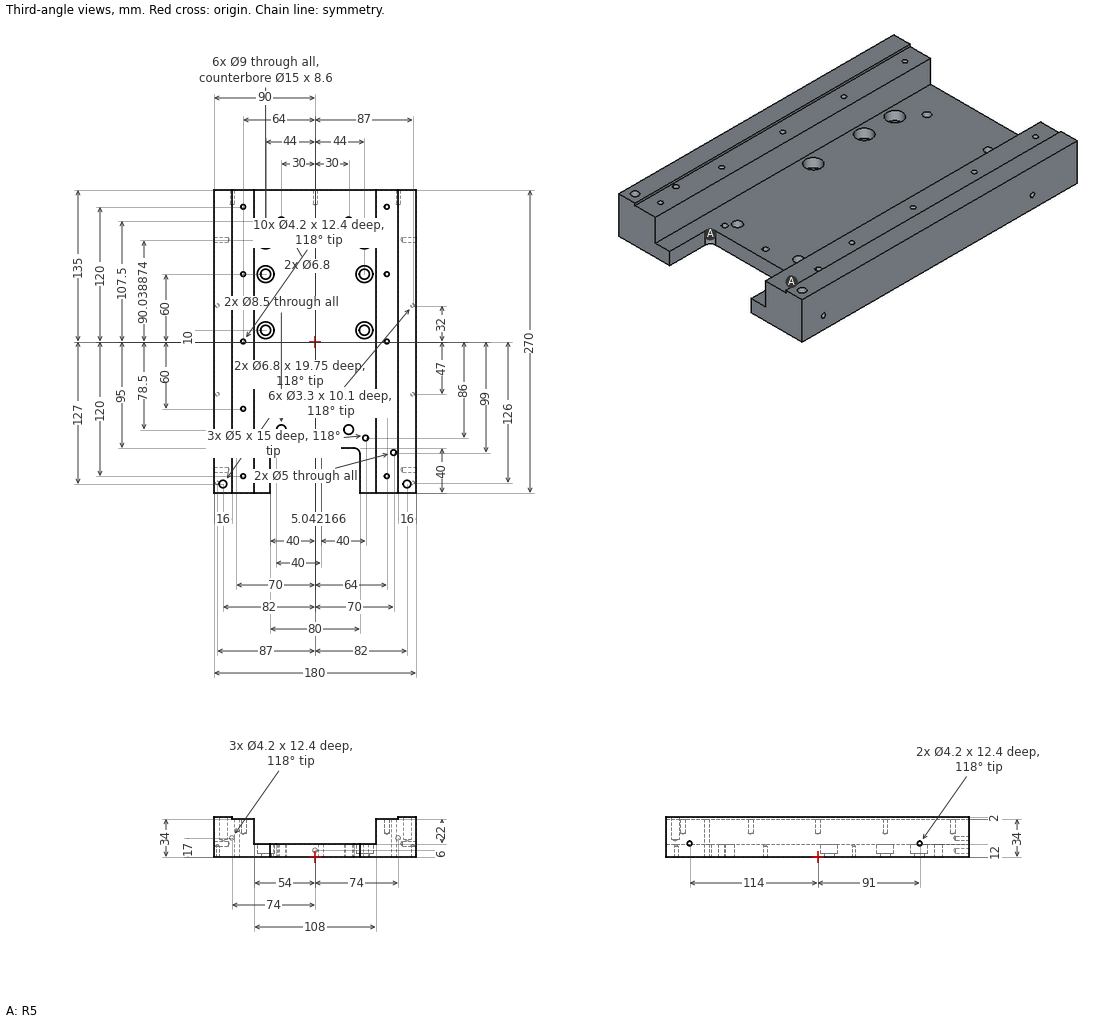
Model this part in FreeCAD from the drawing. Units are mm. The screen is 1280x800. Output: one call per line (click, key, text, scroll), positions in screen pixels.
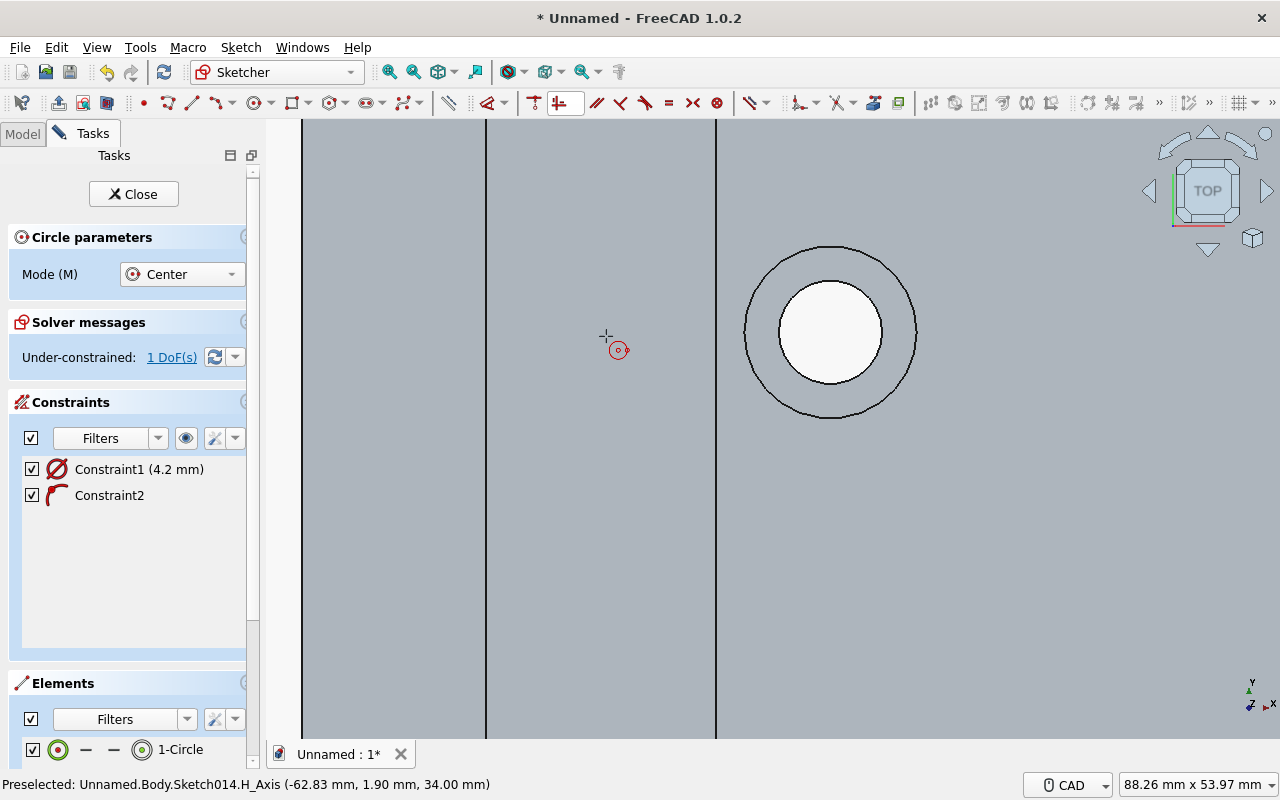
scroll(606, 336, down, 10)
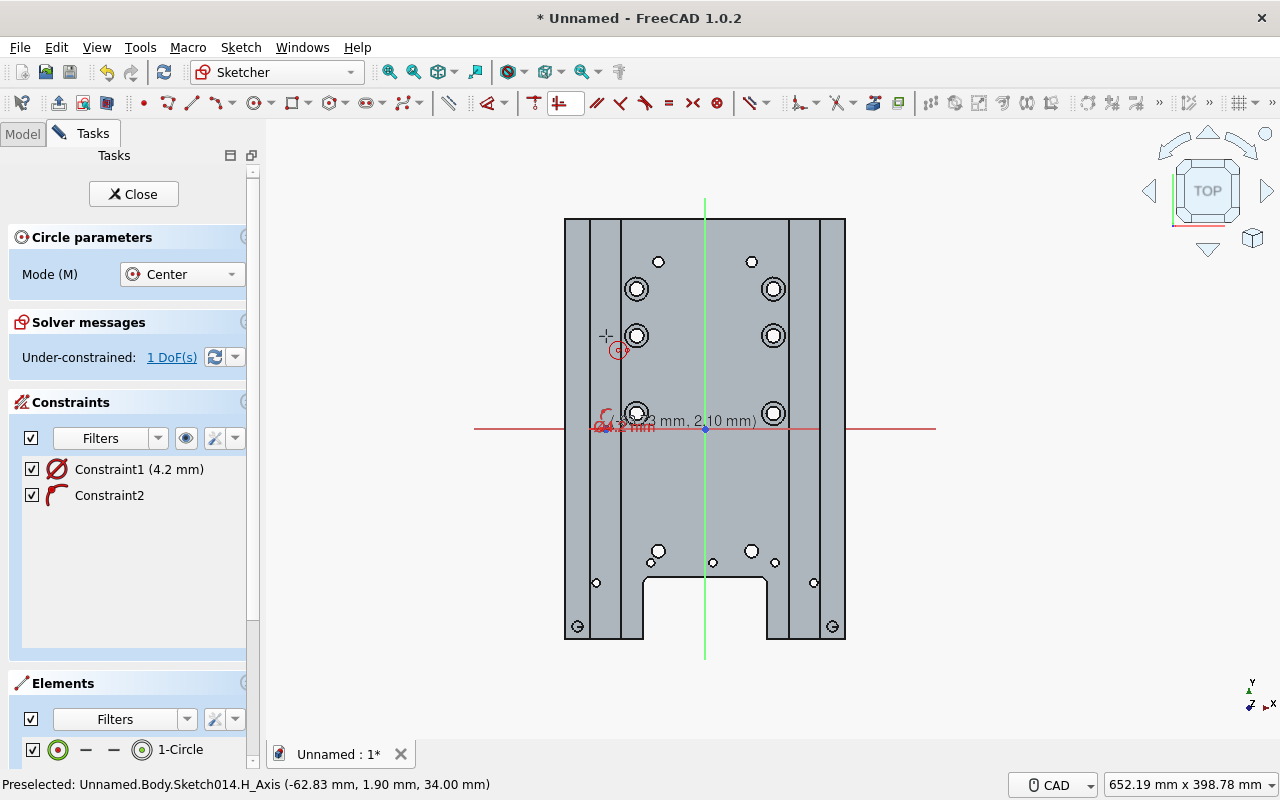
click(606, 336)
move(608, 333)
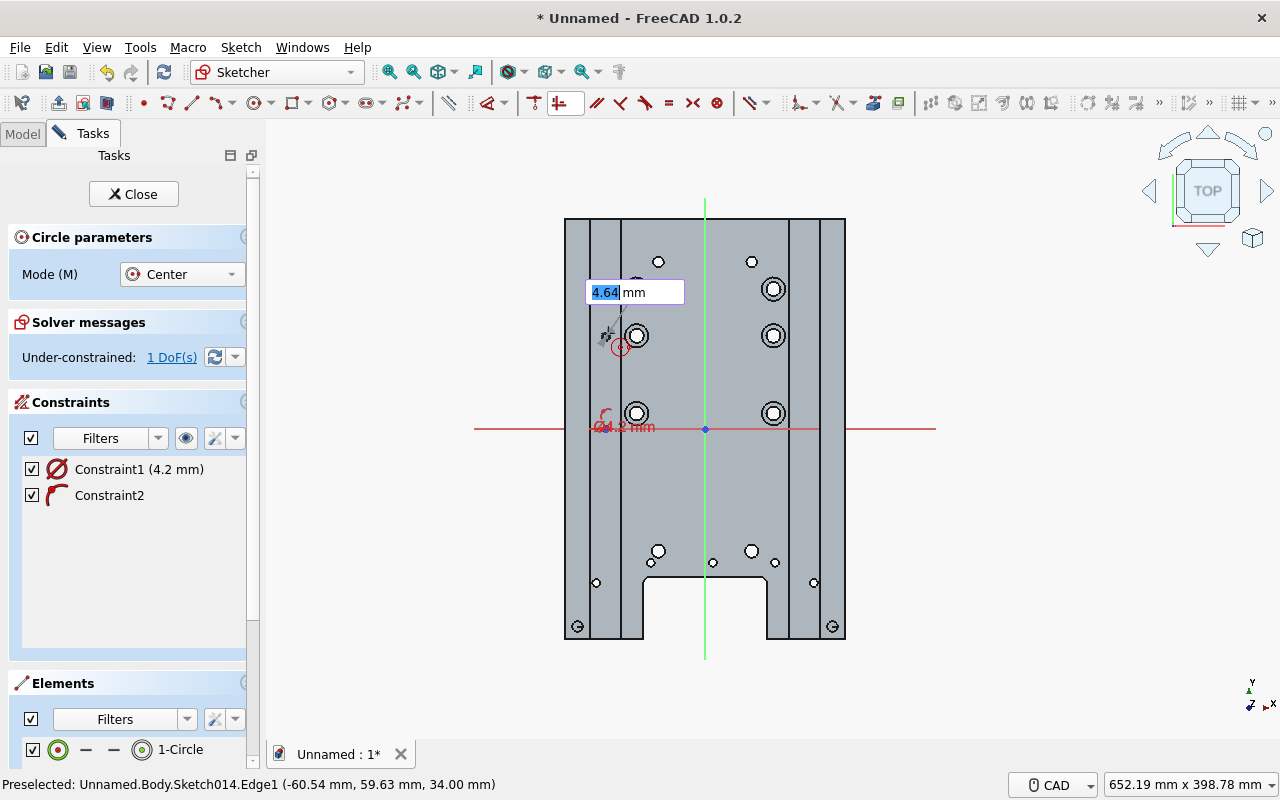
text(4.2)
key(Return)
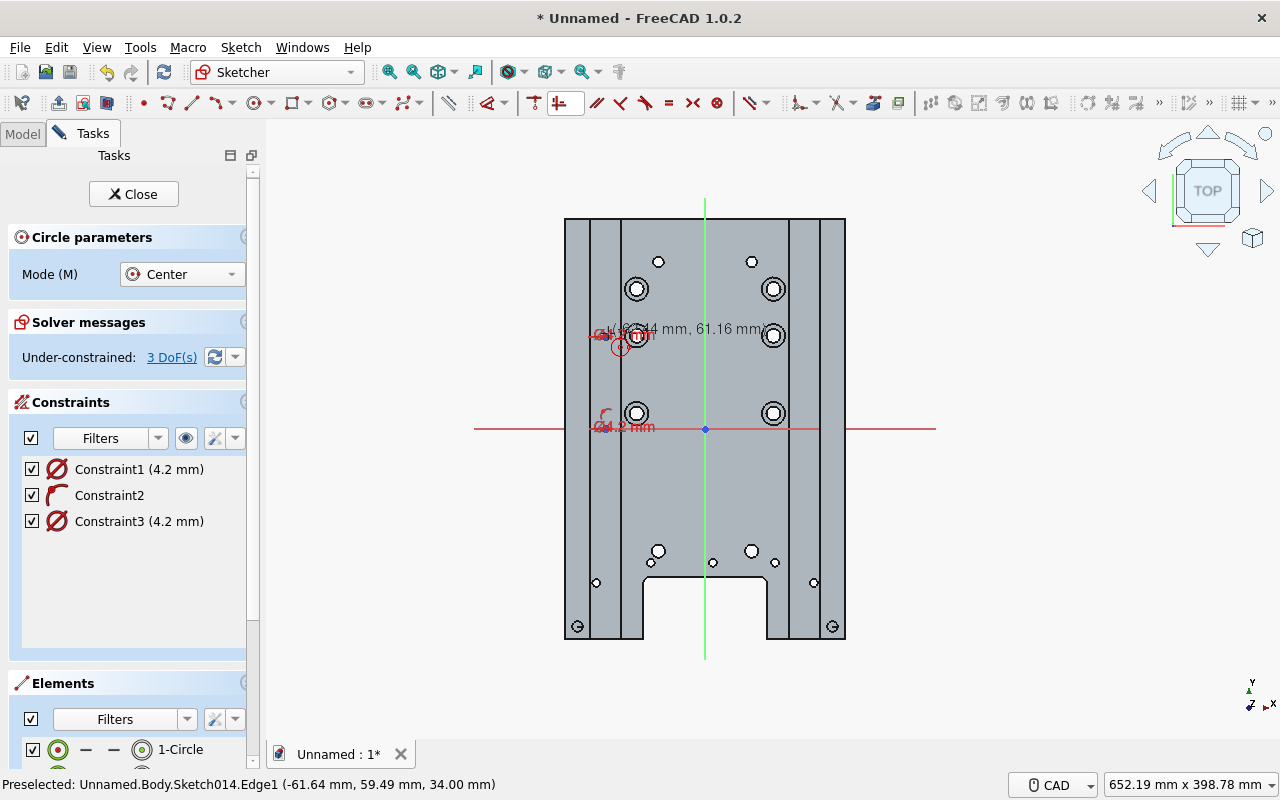
scroll(606, 243, up, 10)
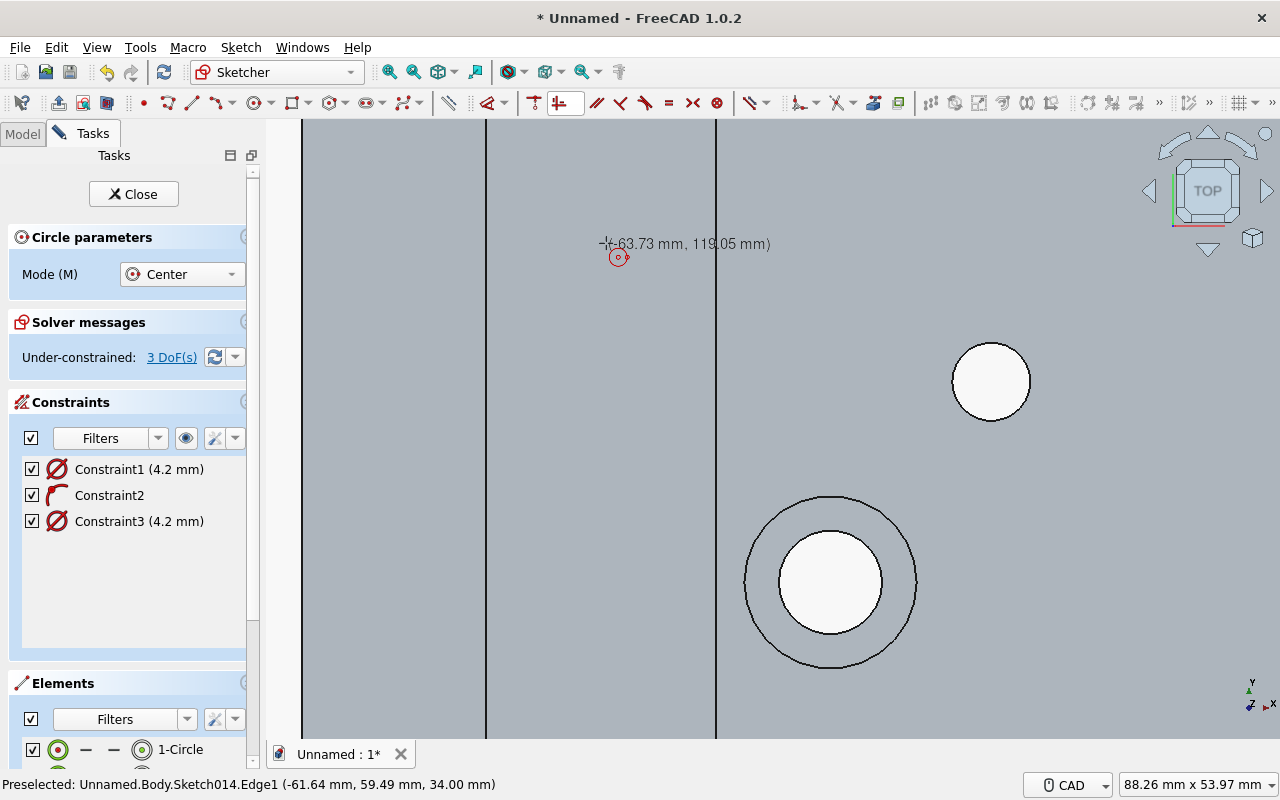
scroll(606, 243, down, 10)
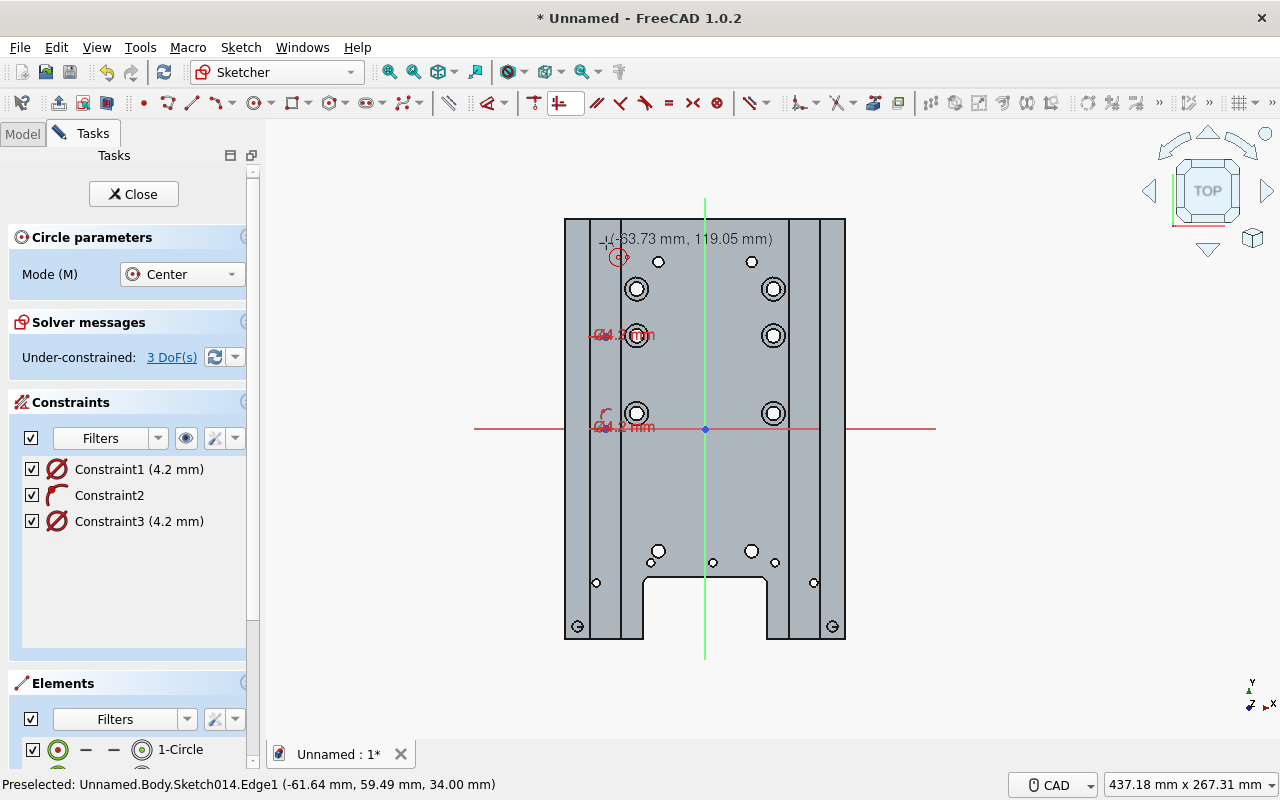
click(606, 243)
move(608, 240)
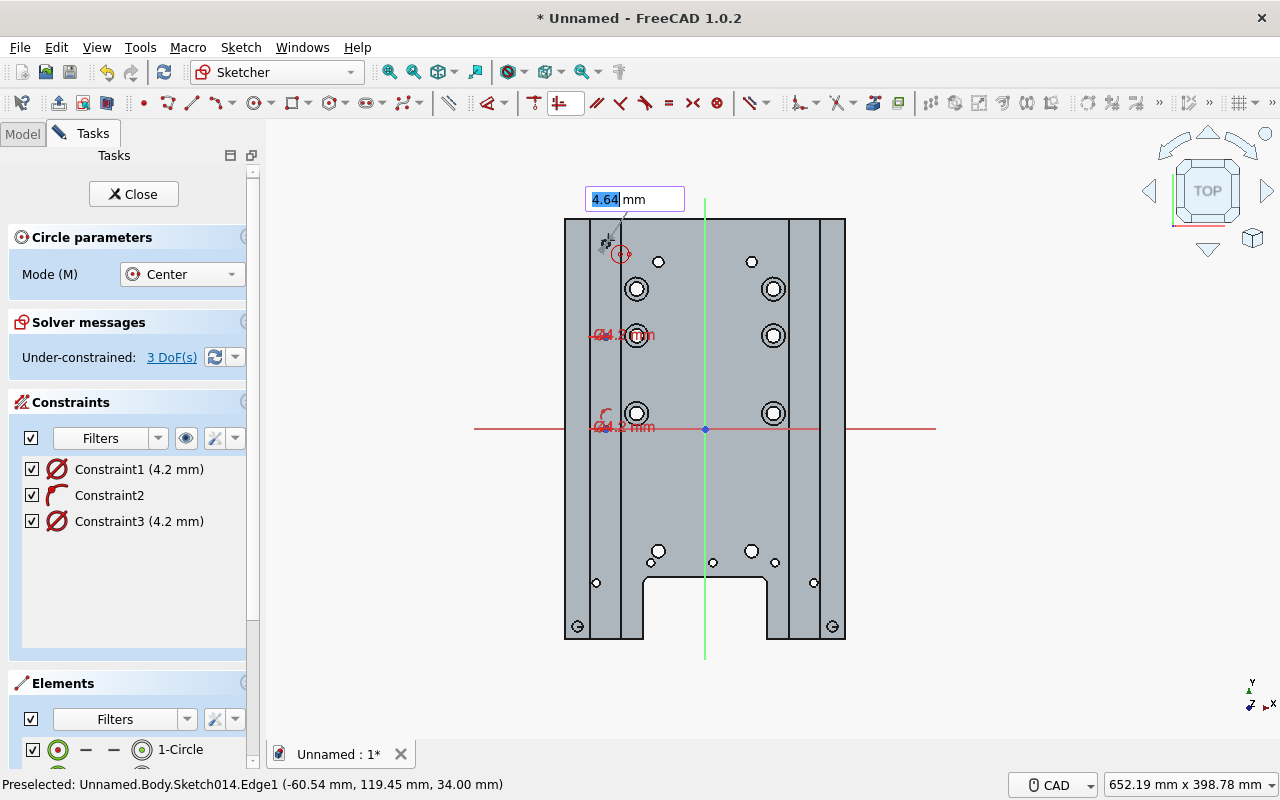
text(4.2)
key(Return)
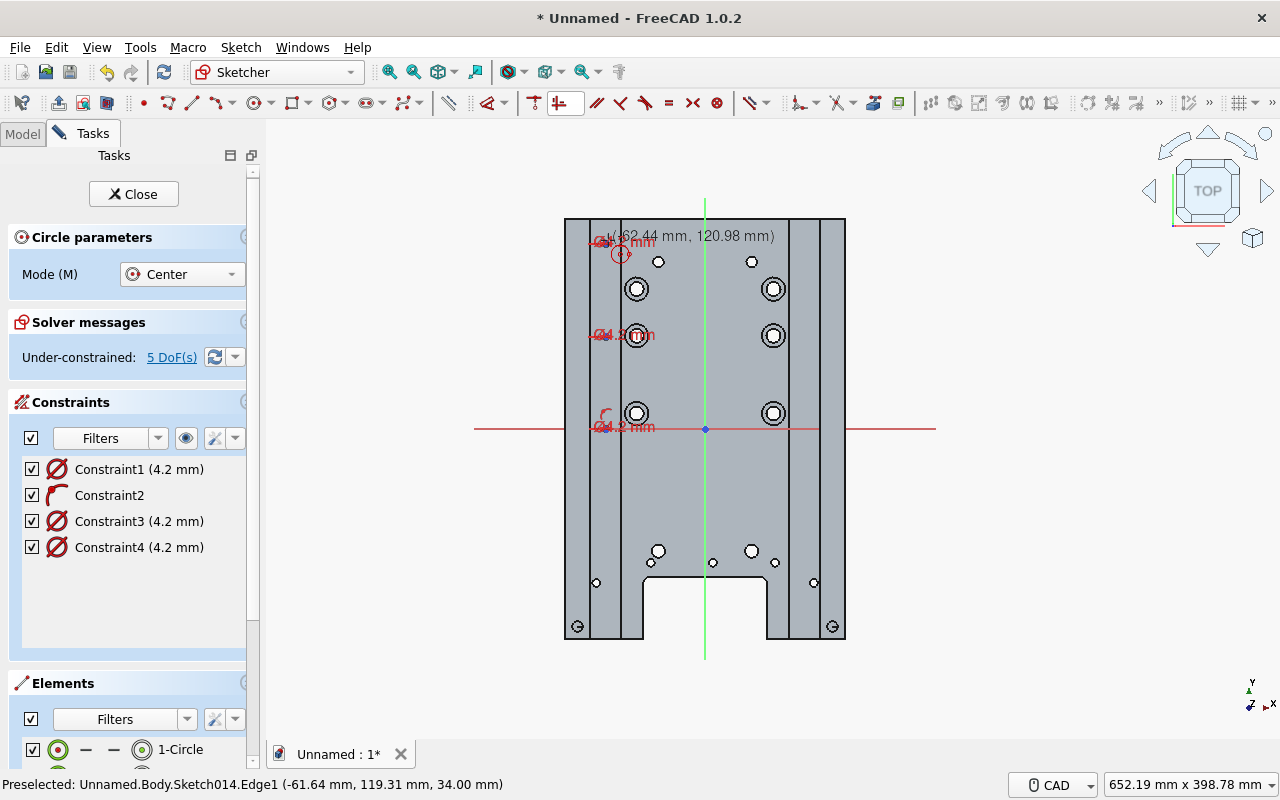
scroll(606, 616, up, 10)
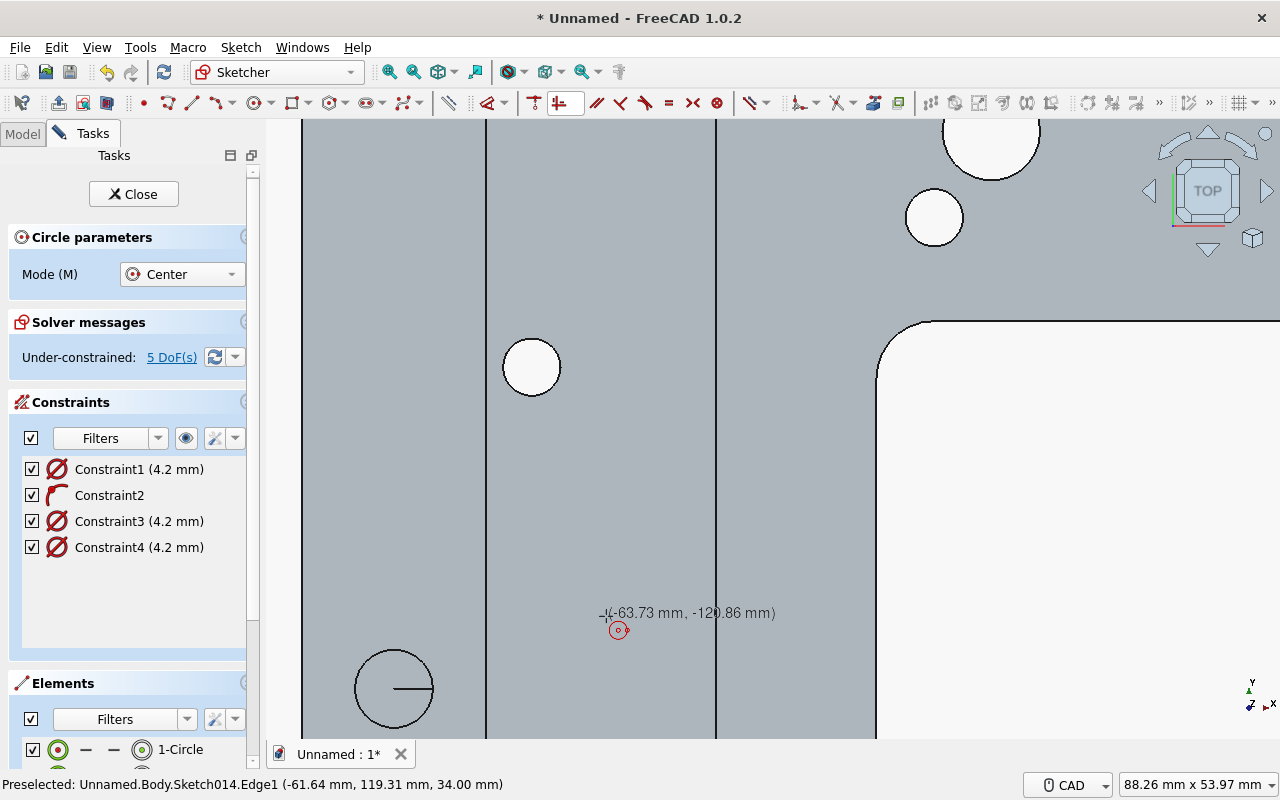
scroll(606, 617, down, 10)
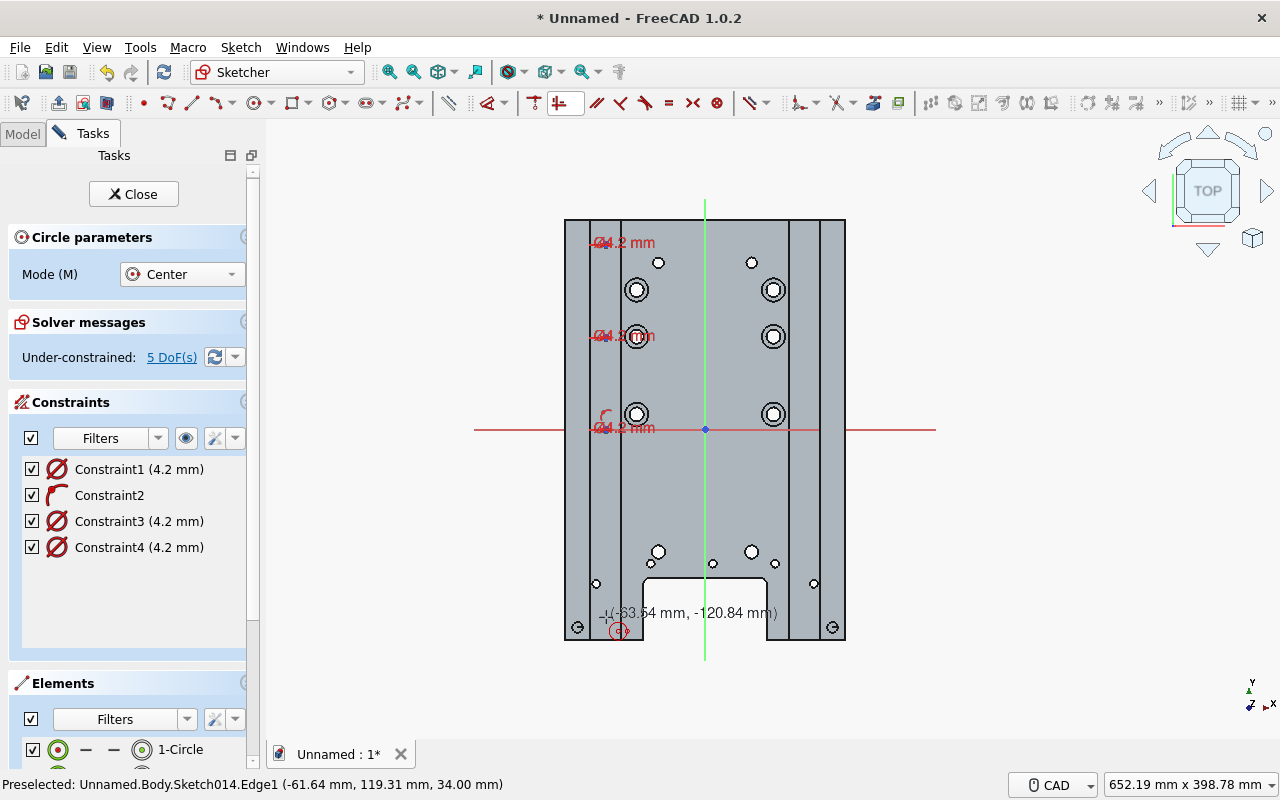
click(606, 617)
move(608, 614)